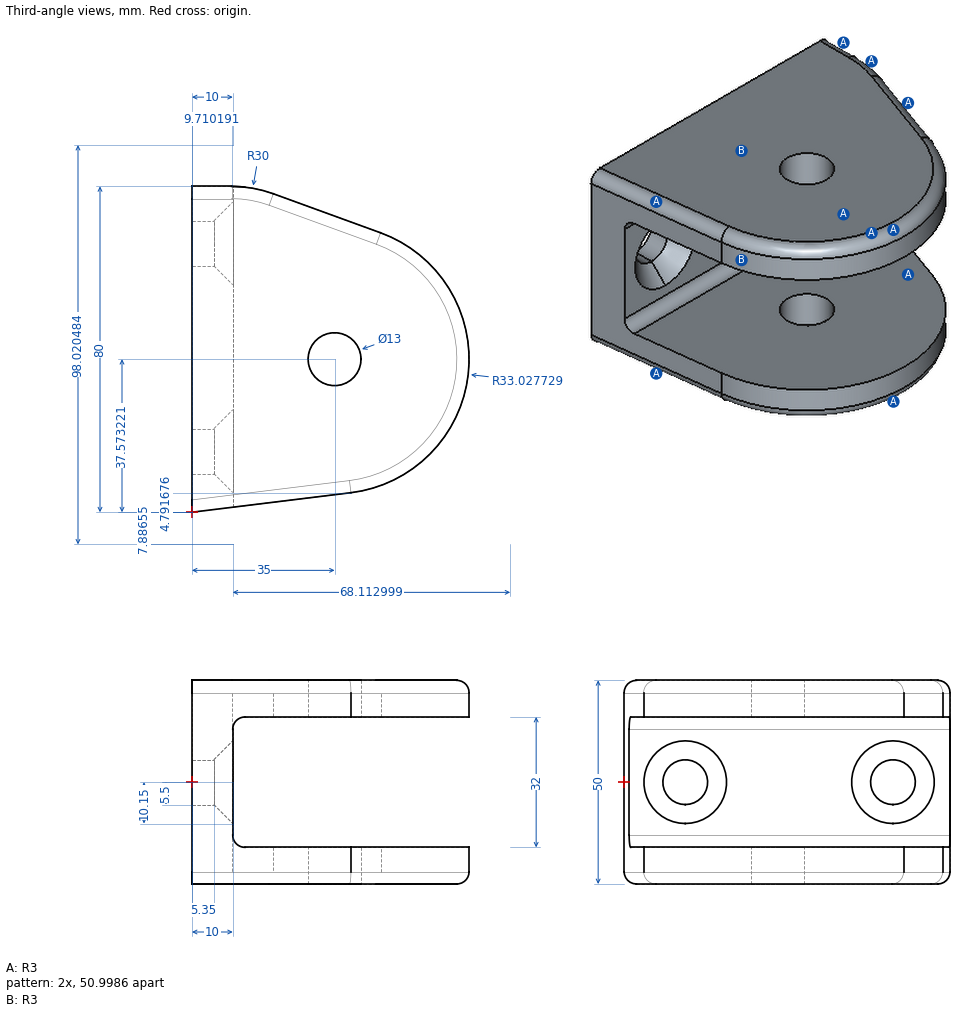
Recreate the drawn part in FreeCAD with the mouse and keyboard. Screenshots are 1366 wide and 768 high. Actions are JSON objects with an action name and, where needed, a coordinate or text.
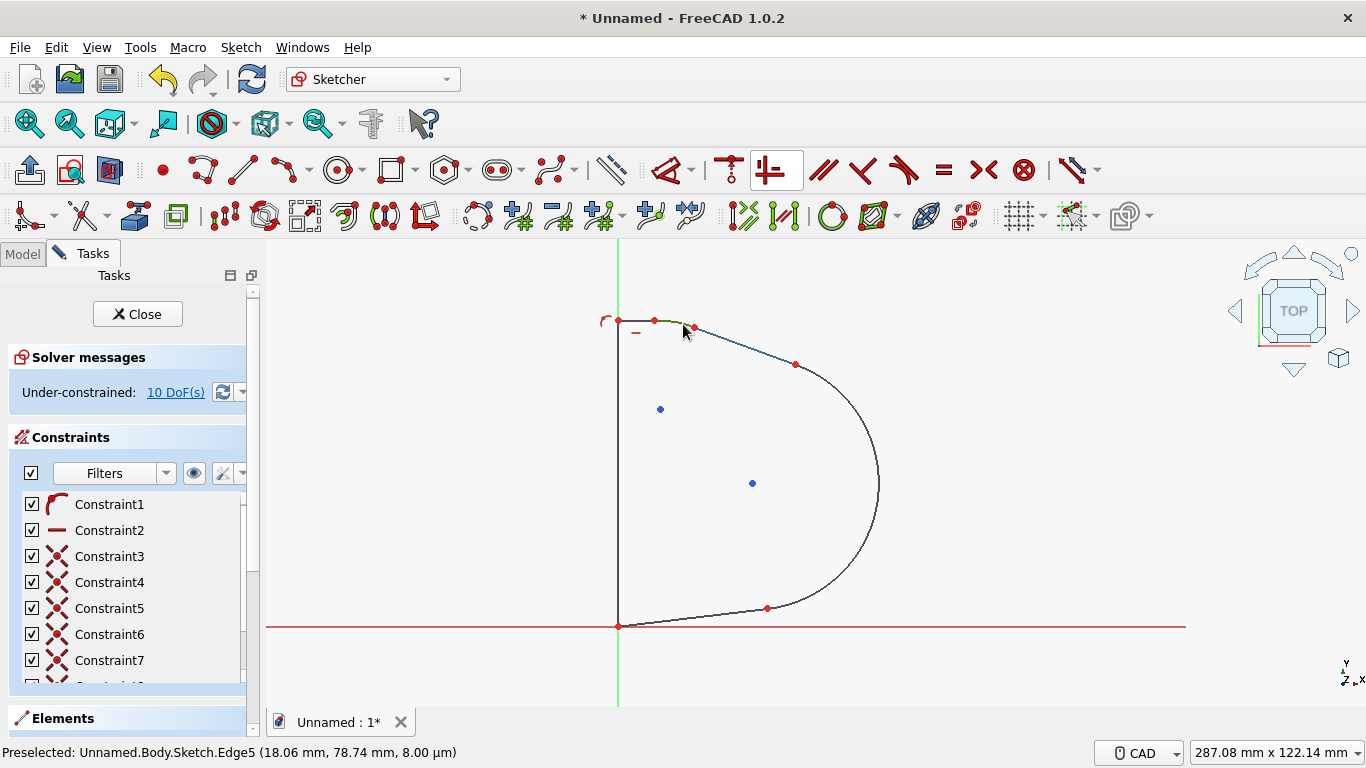
{"action": "left_click", "coordinate": [904, 170]}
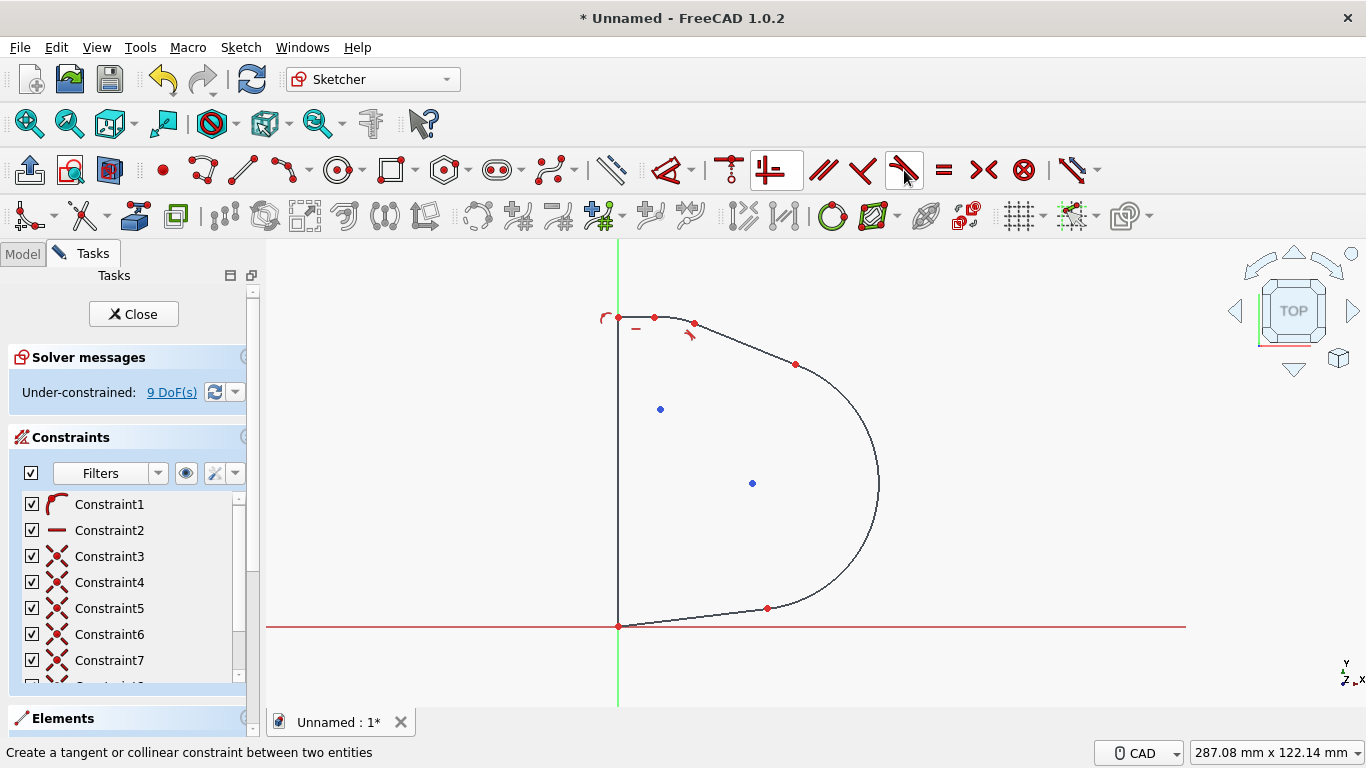
{"action": "left_click", "coordinate": [766, 353]}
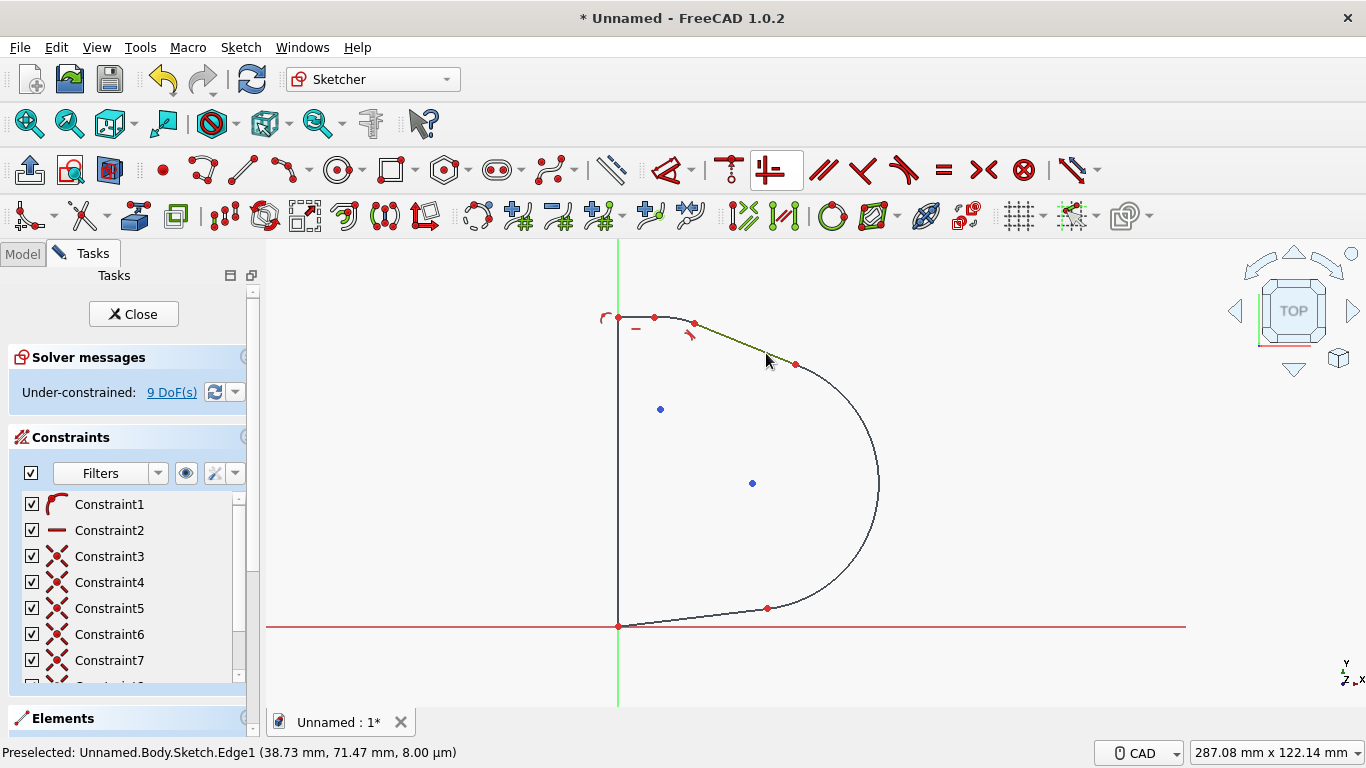
{"action": "left_click", "coordinate": [853, 560]}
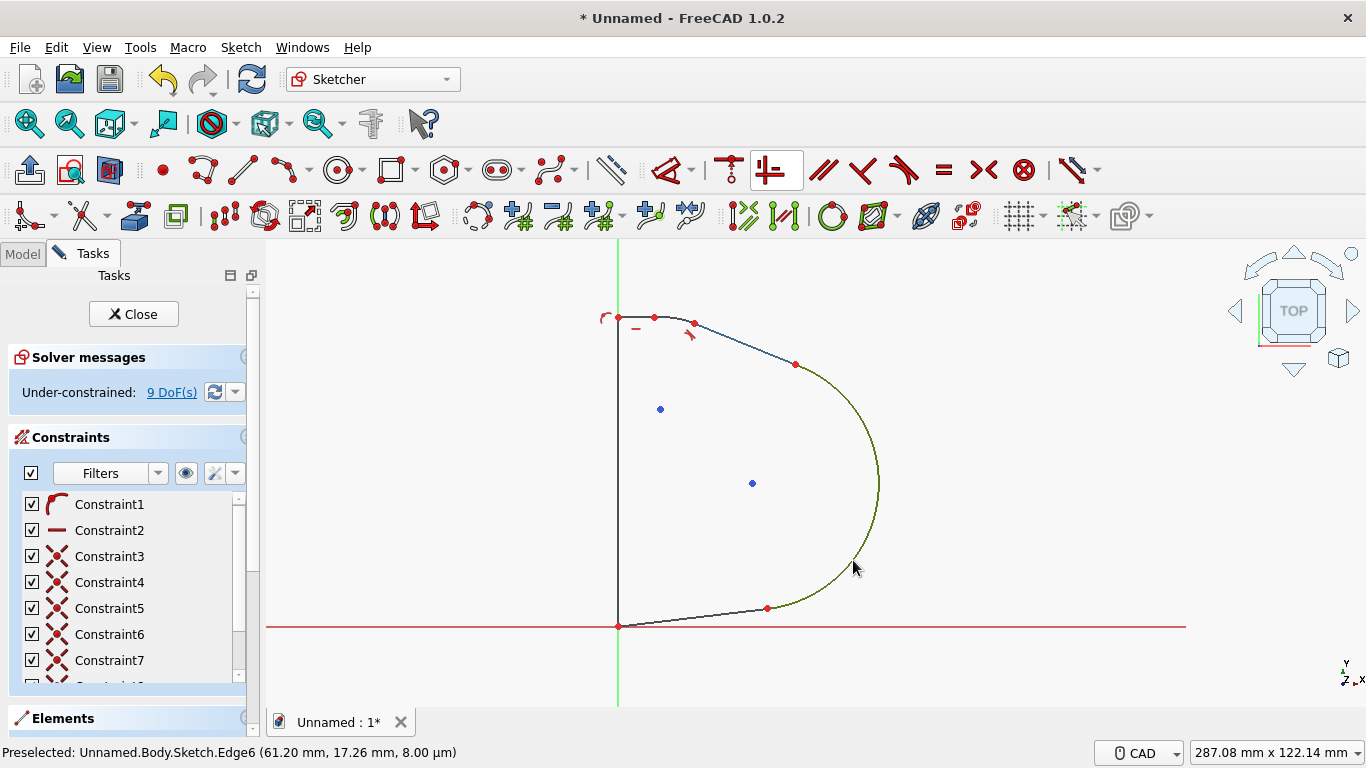
{"action": "left_click", "coordinate": [904, 170]}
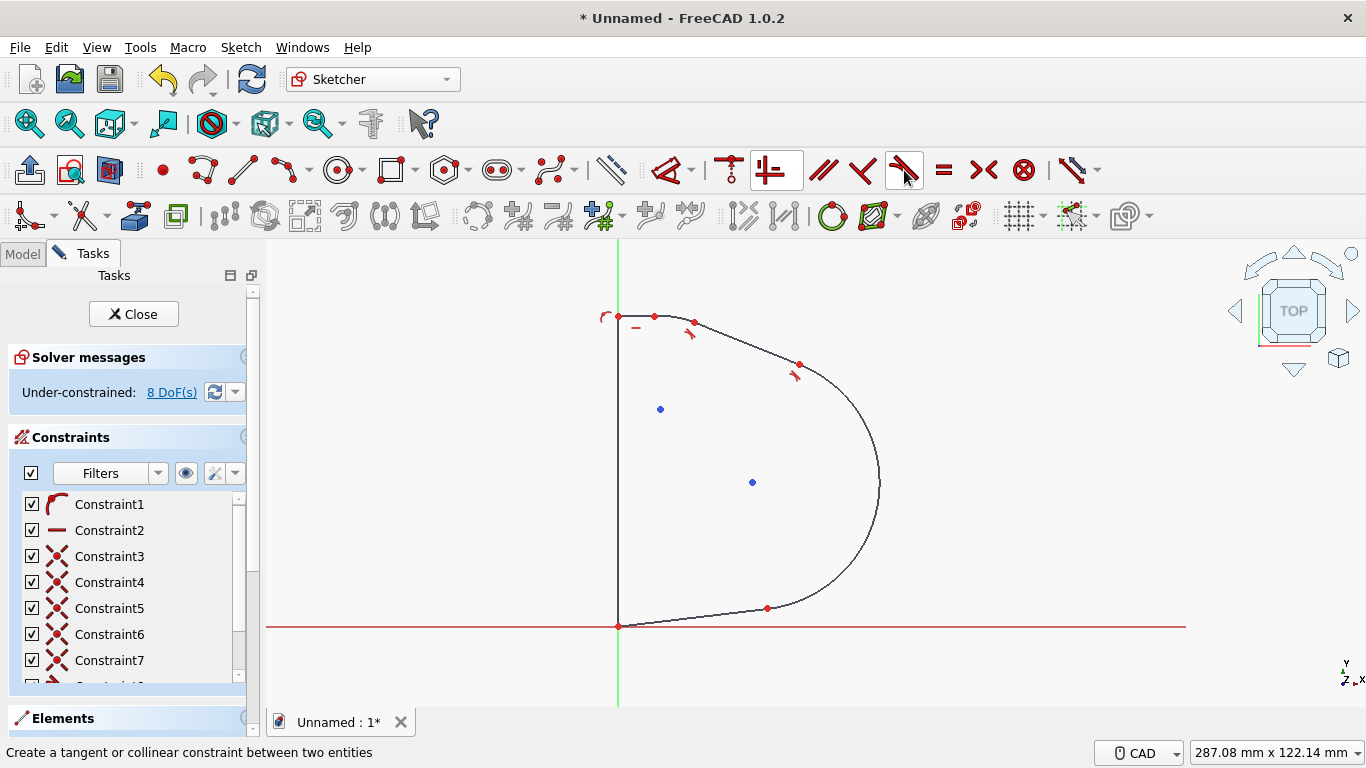
{"action": "scroll", "coordinate": [644, 316], "scroll_direction": "up", "scroll_amount": 2}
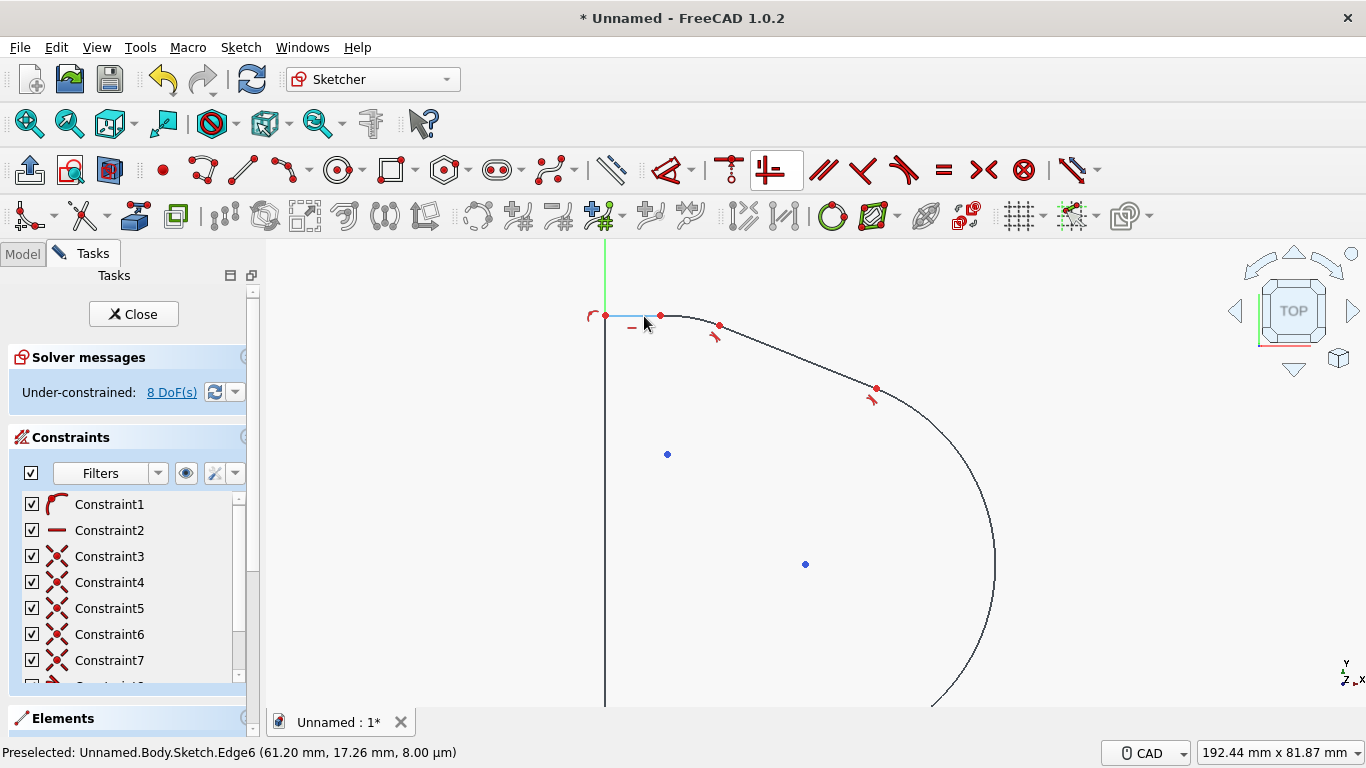
{"action": "left_click", "coordinate": [644, 316]}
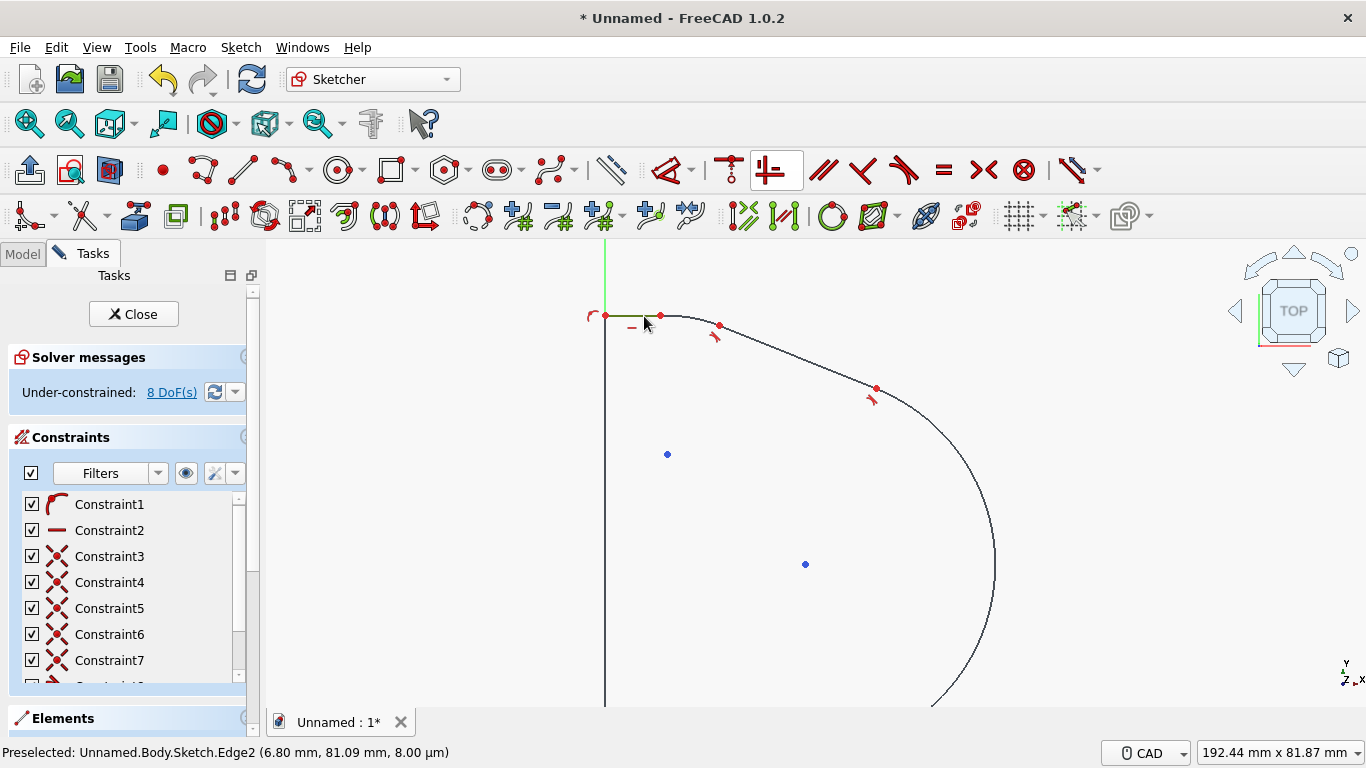
{"action": "left_click", "coordinate": [702, 320]}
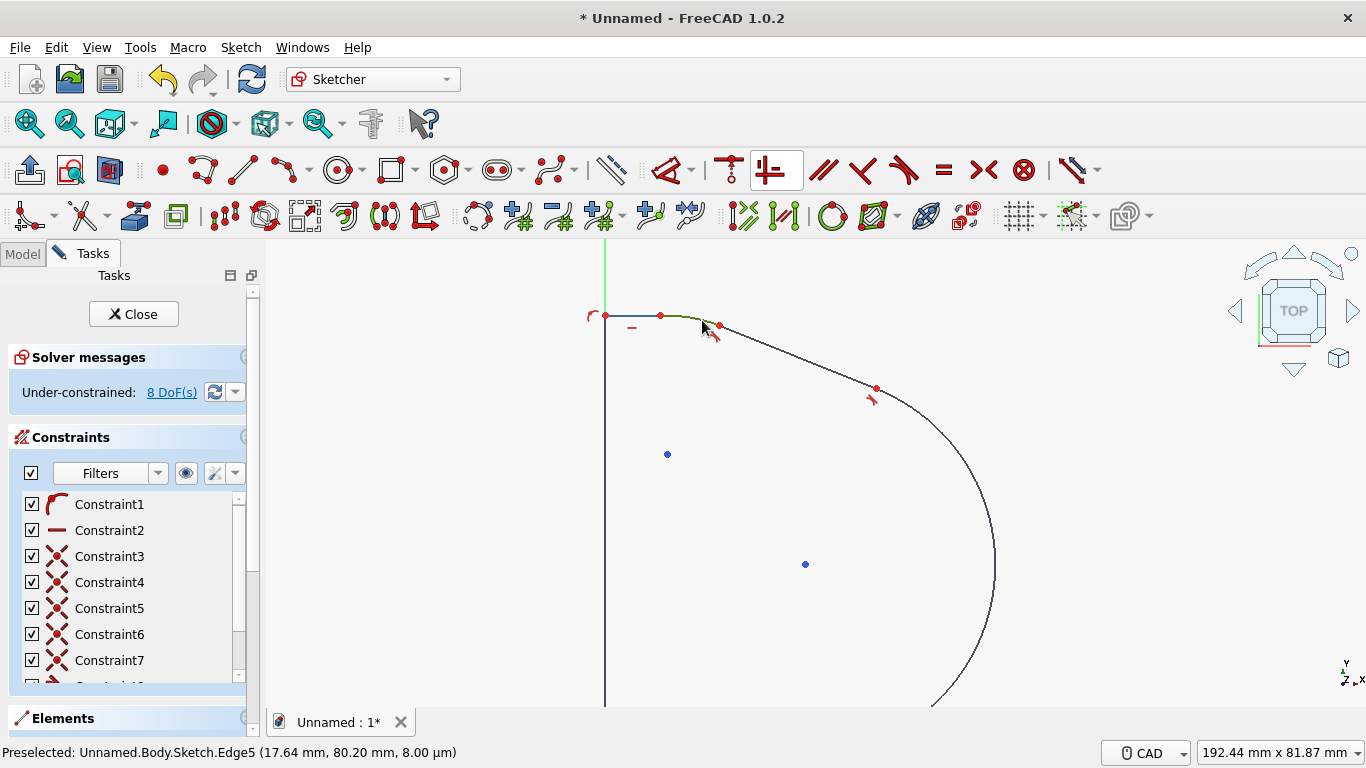
{"action": "left_click", "coordinate": [904, 170]}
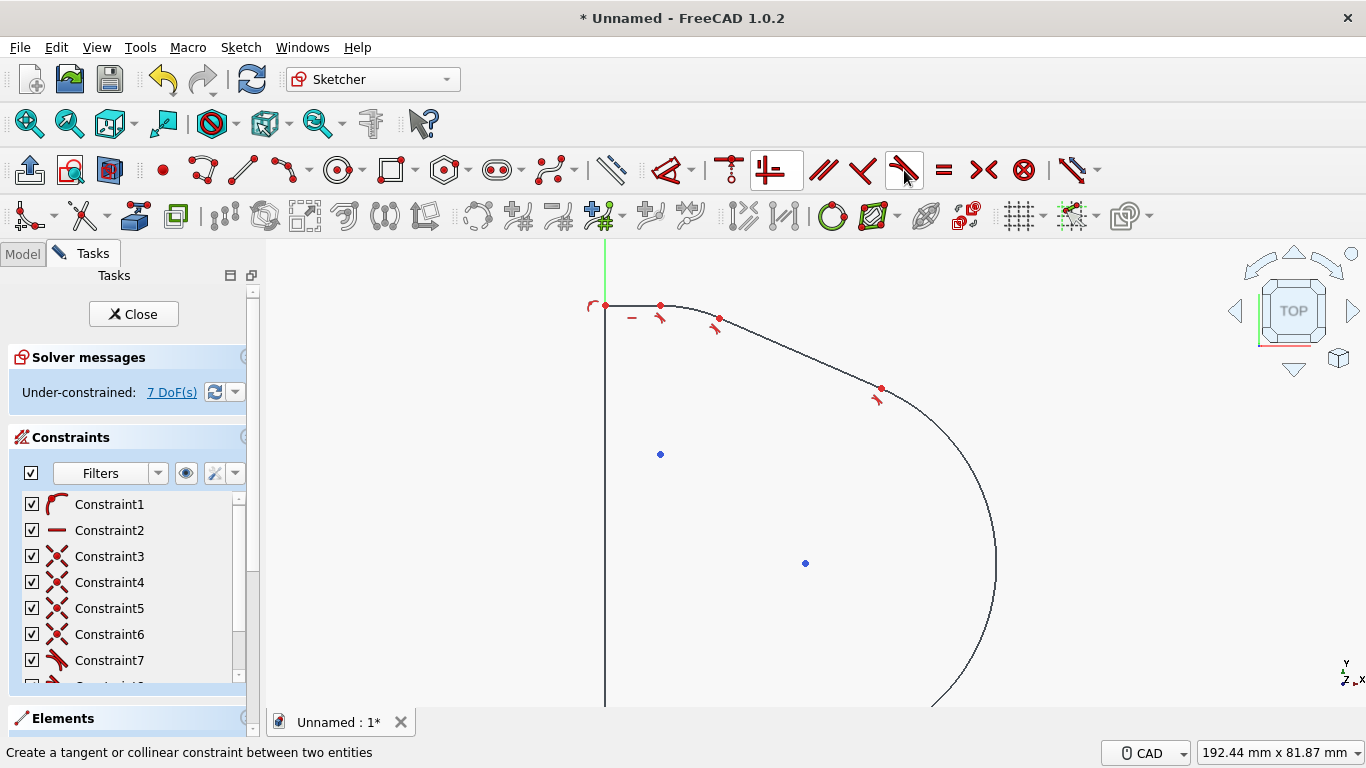
{"action": "scroll", "coordinate": [643, 315], "scroll_direction": "down", "scroll_amount": 2}